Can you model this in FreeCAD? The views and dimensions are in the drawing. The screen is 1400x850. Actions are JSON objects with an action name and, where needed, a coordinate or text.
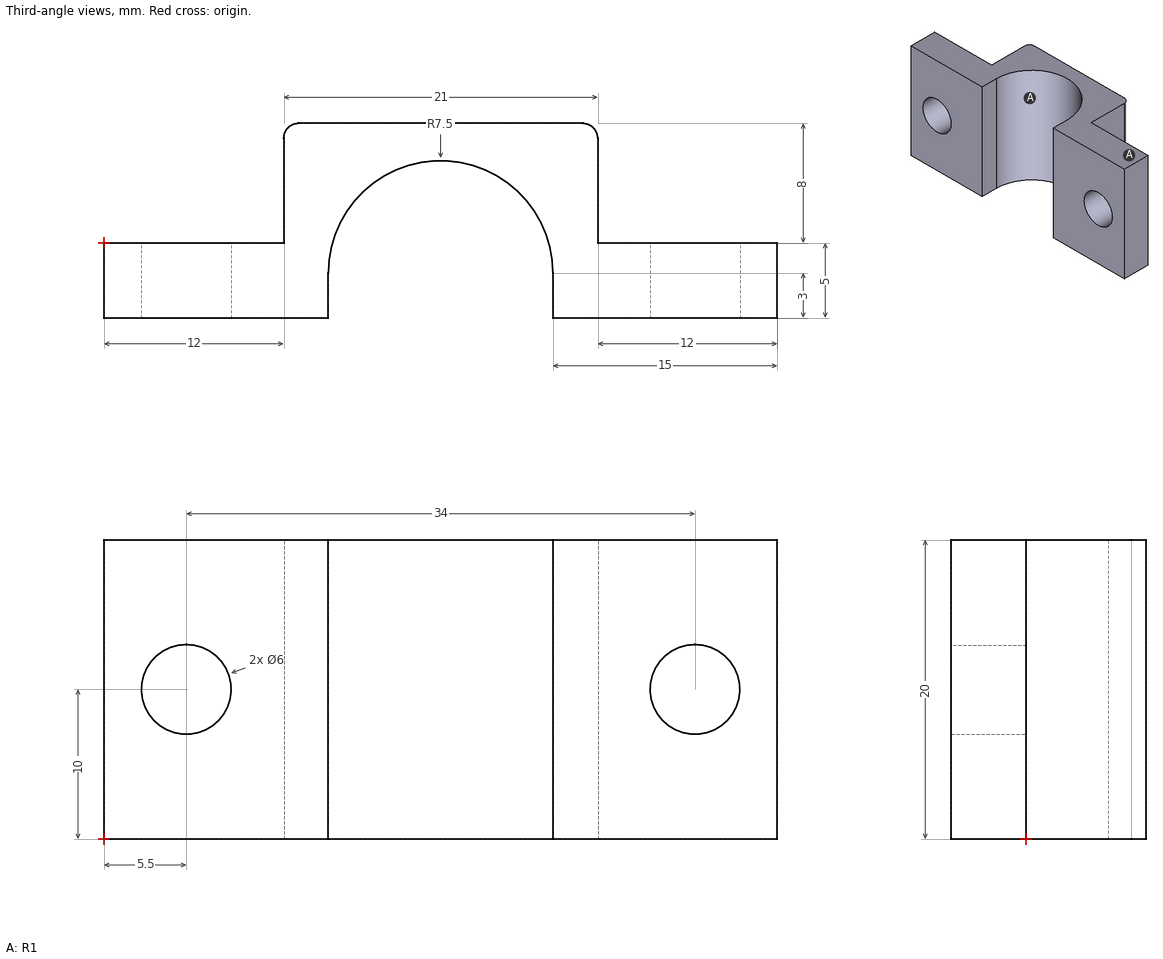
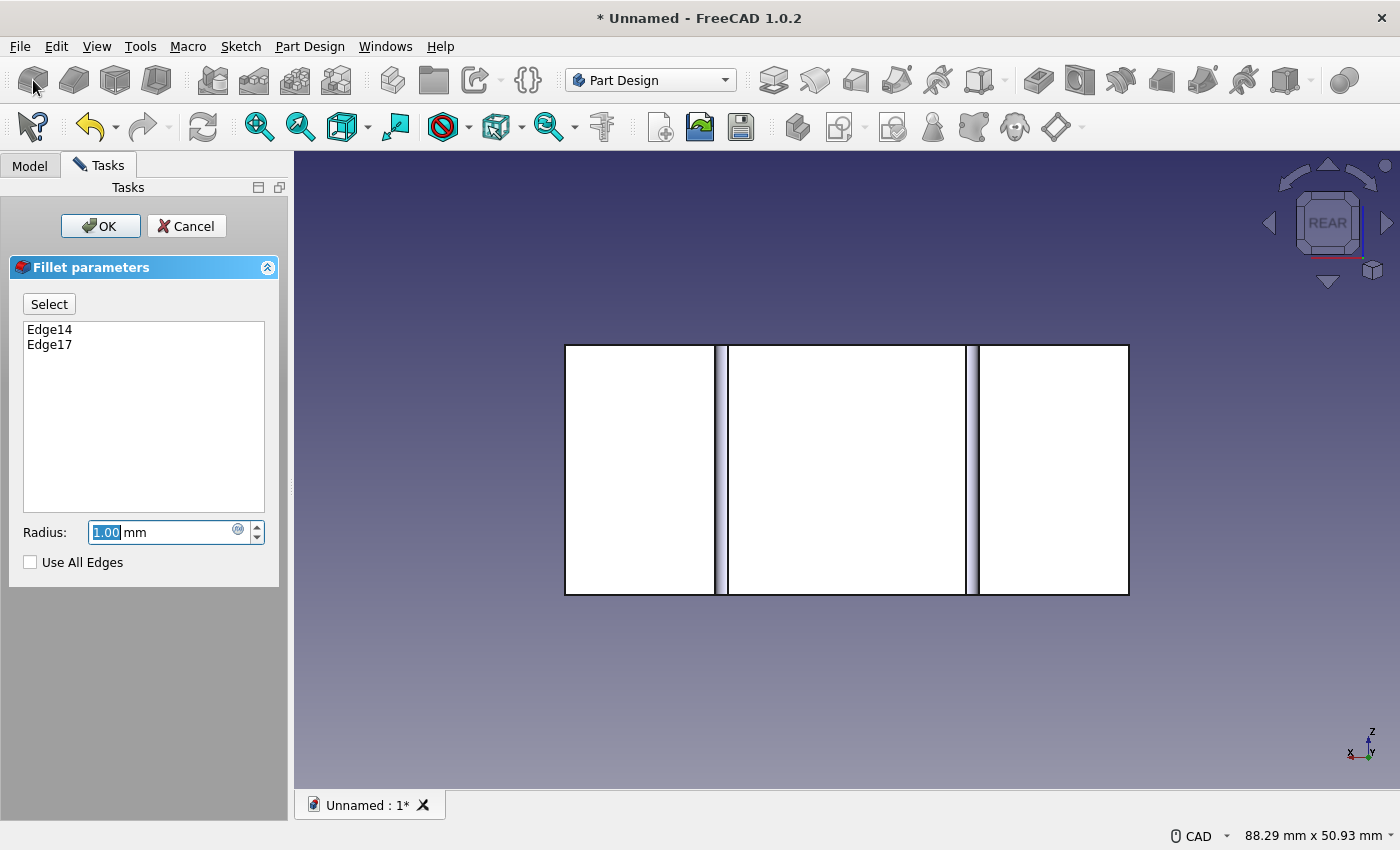
{"action": "type", "text": "1"}
{"action": "key", "text": "Tab"}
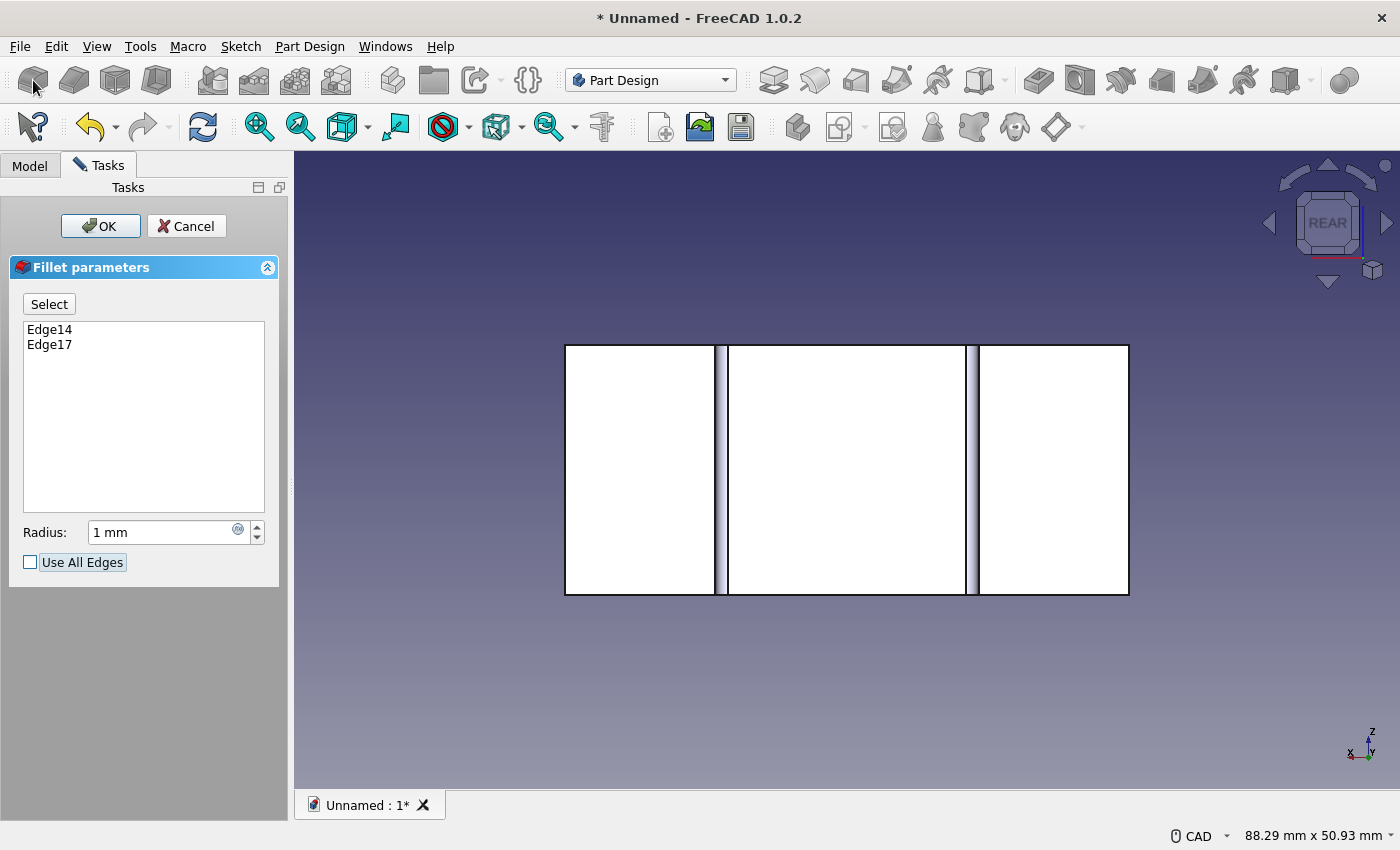
{"action": "left_click", "coordinate": [101, 226]}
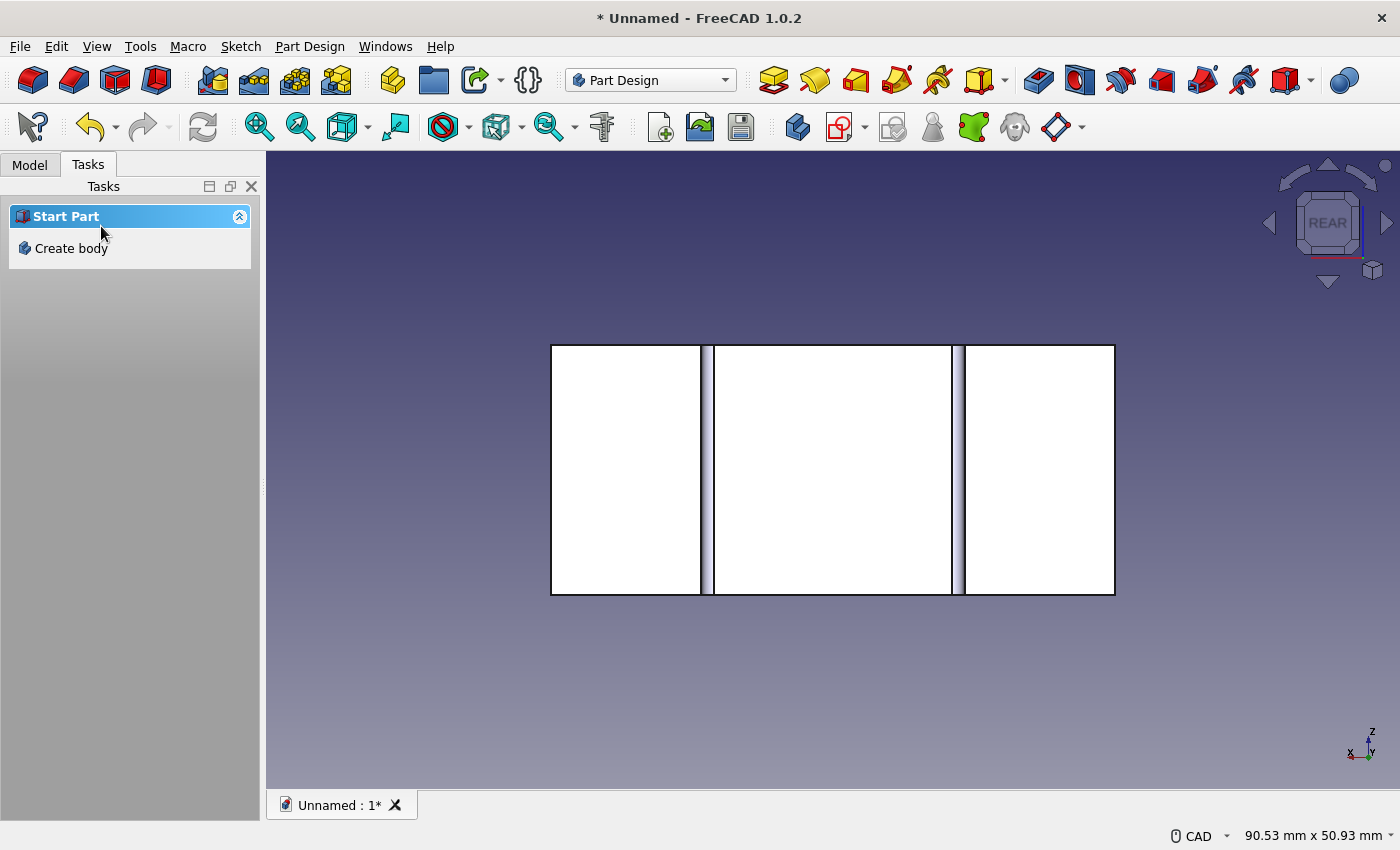
{"action": "left_click", "coordinate": [838, 128]}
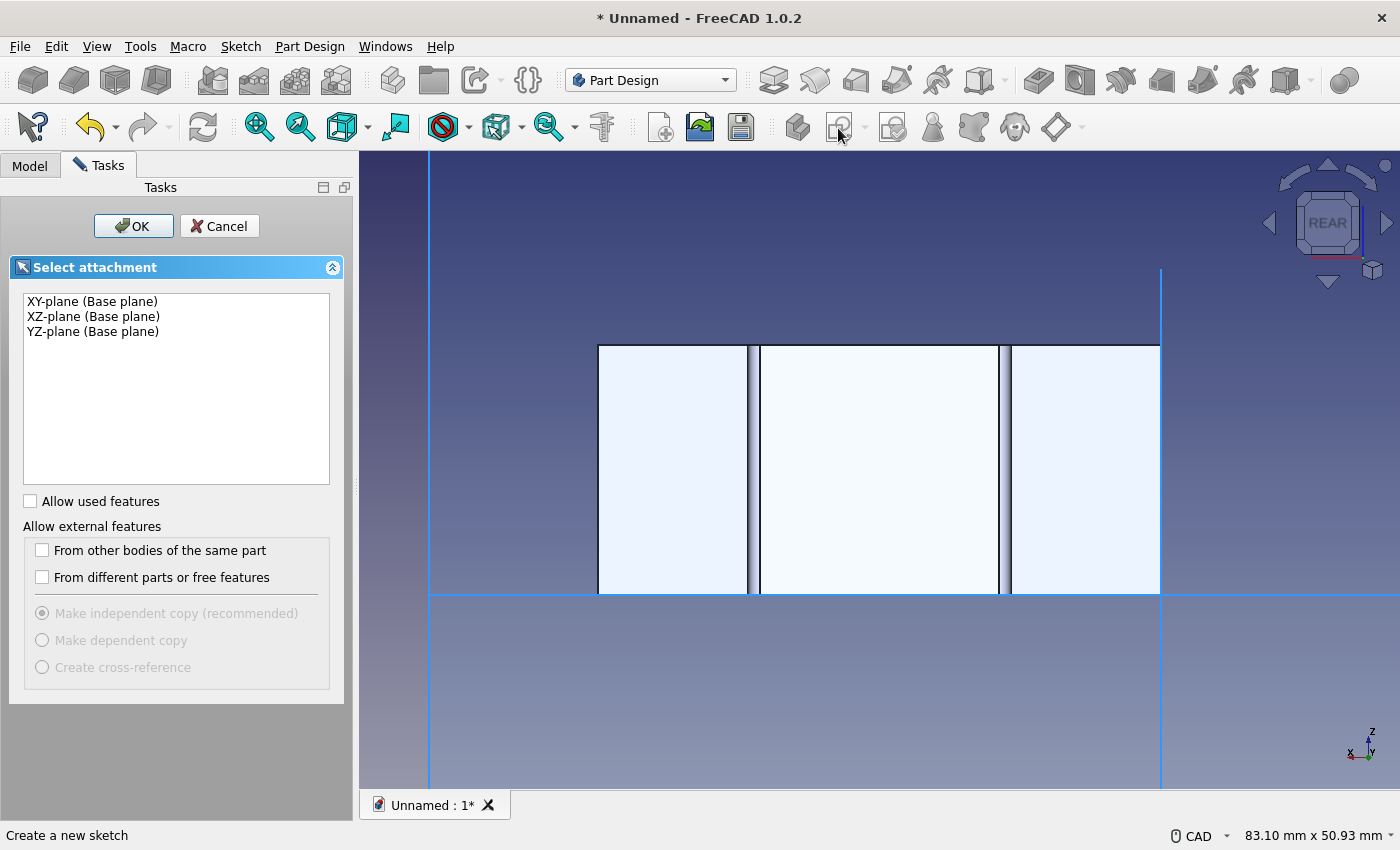
{"action": "left_click", "coordinate": [84, 316]}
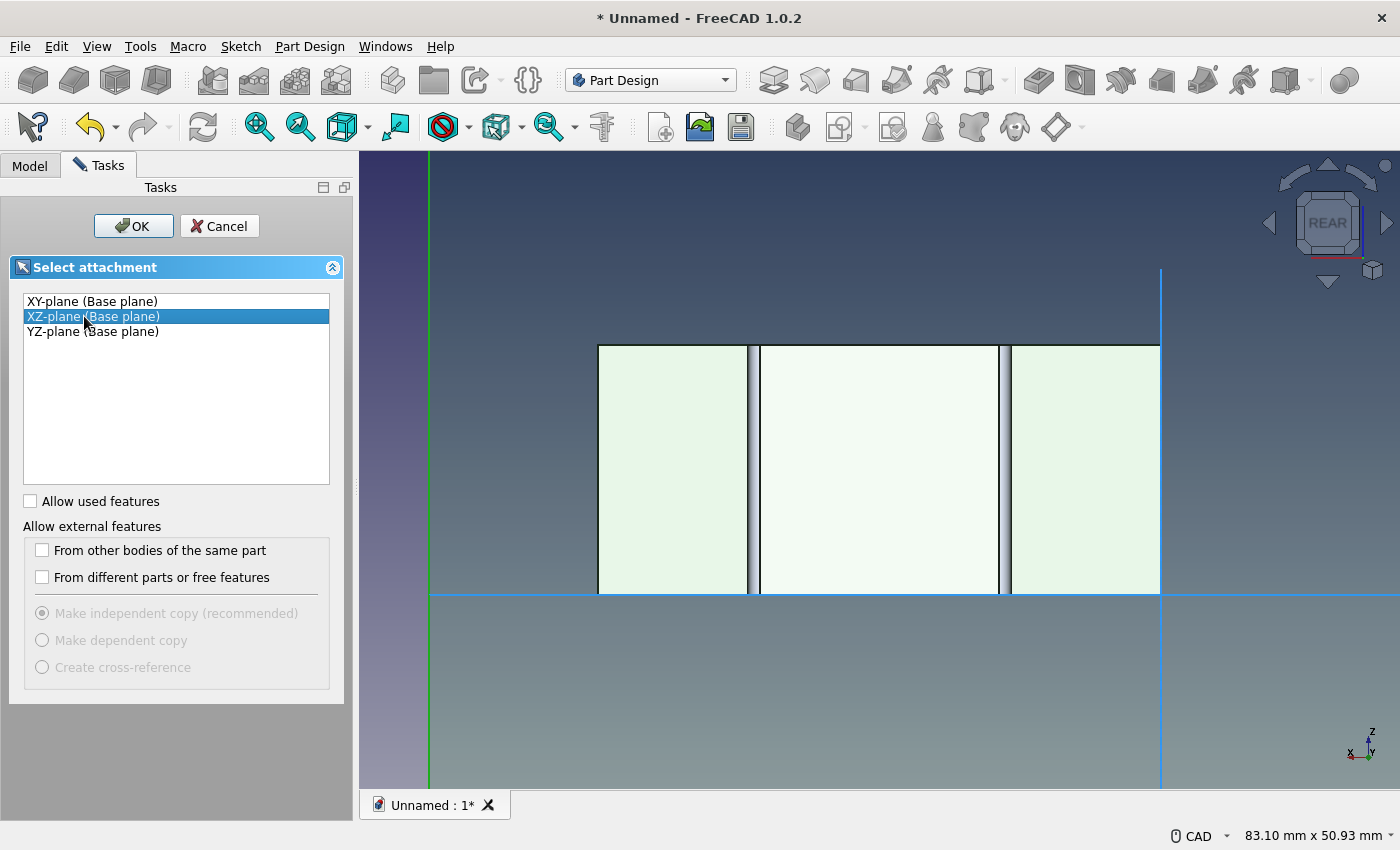
{"action": "left_click", "coordinate": [134, 226]}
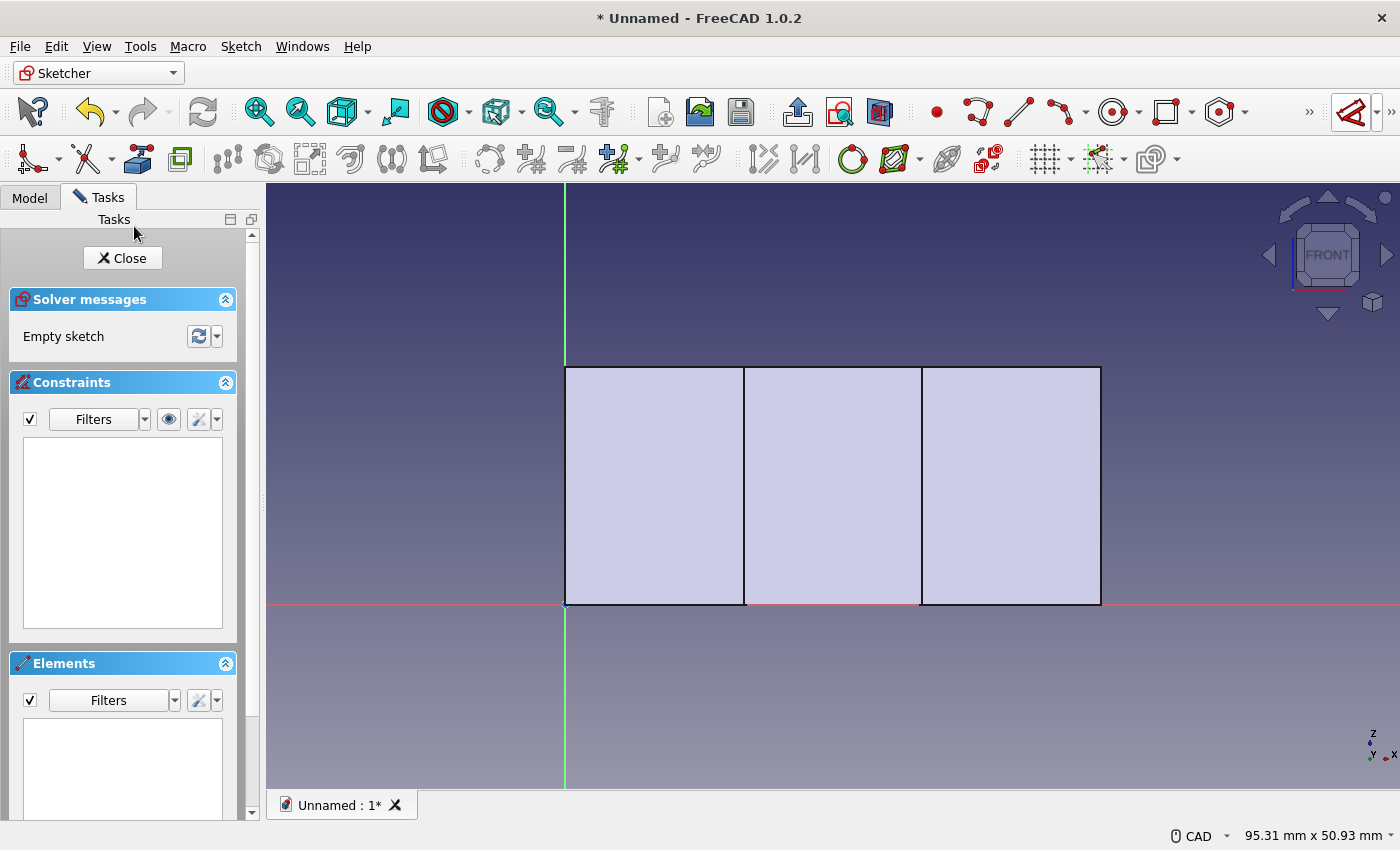
{"action": "left_click", "coordinate": [880, 112]}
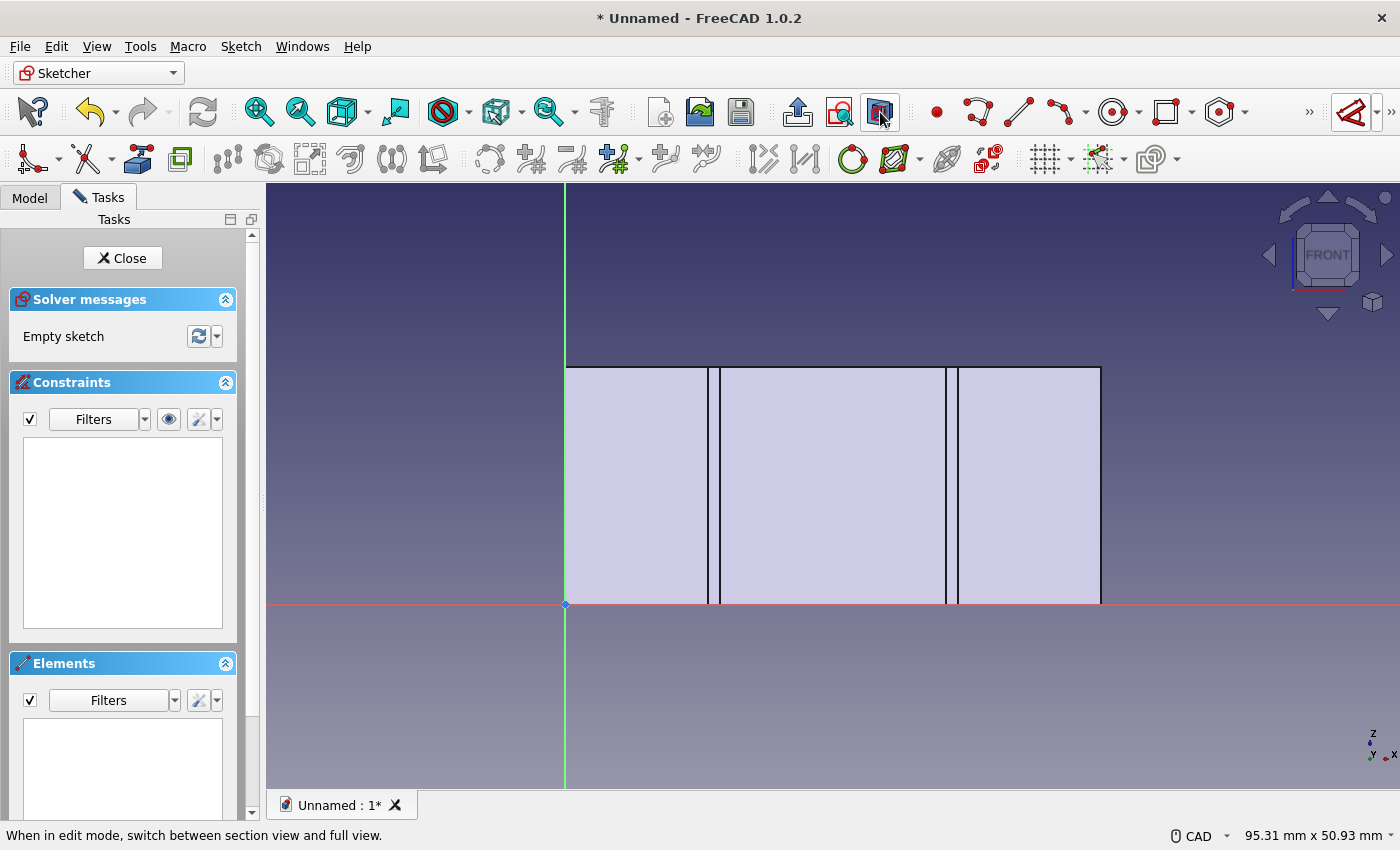
{"action": "left_click", "coordinate": [1112, 112]}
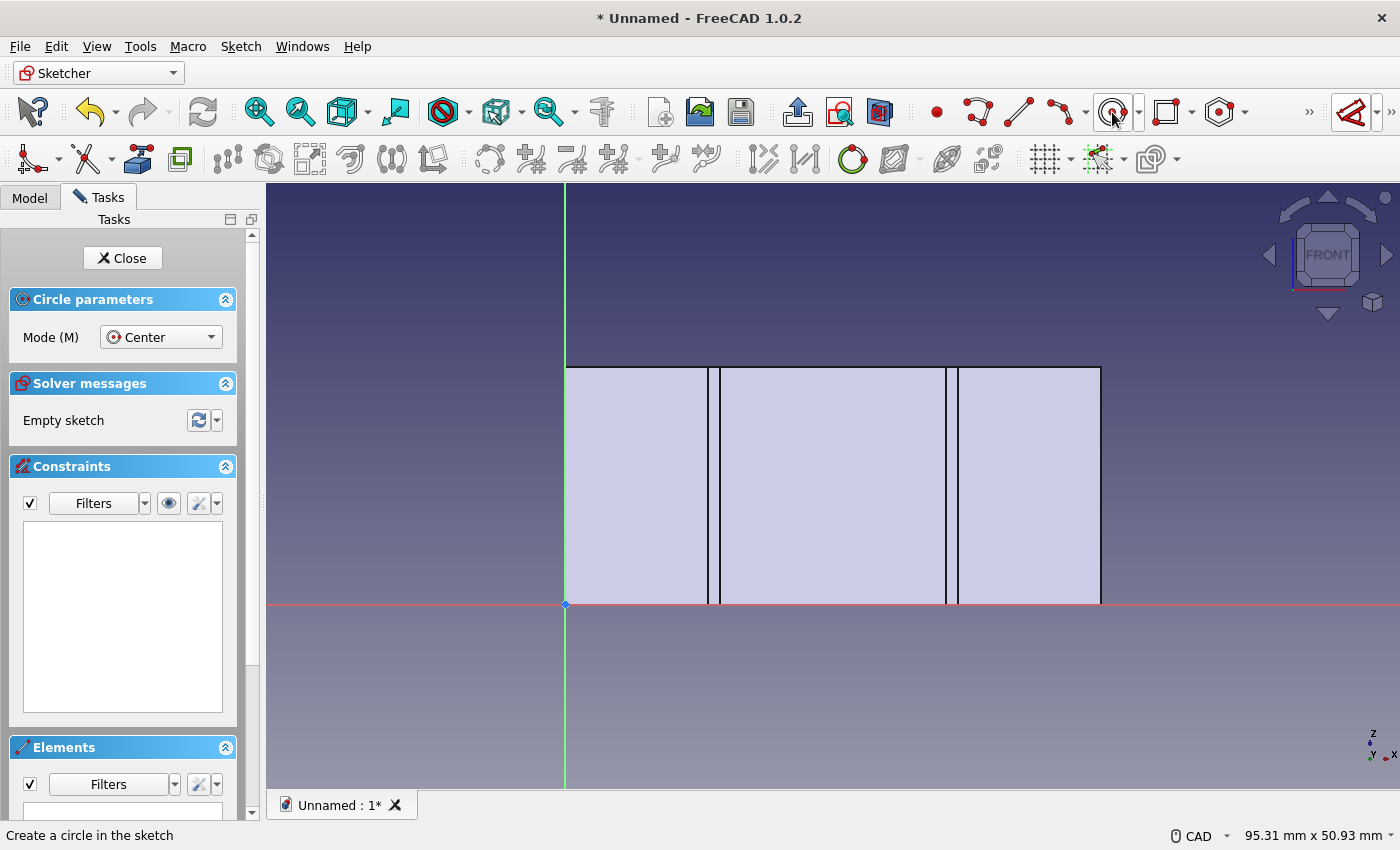
{"action": "left_click", "coordinate": [631, 486]}
{"action": "left_click", "coordinate": [656, 461]}